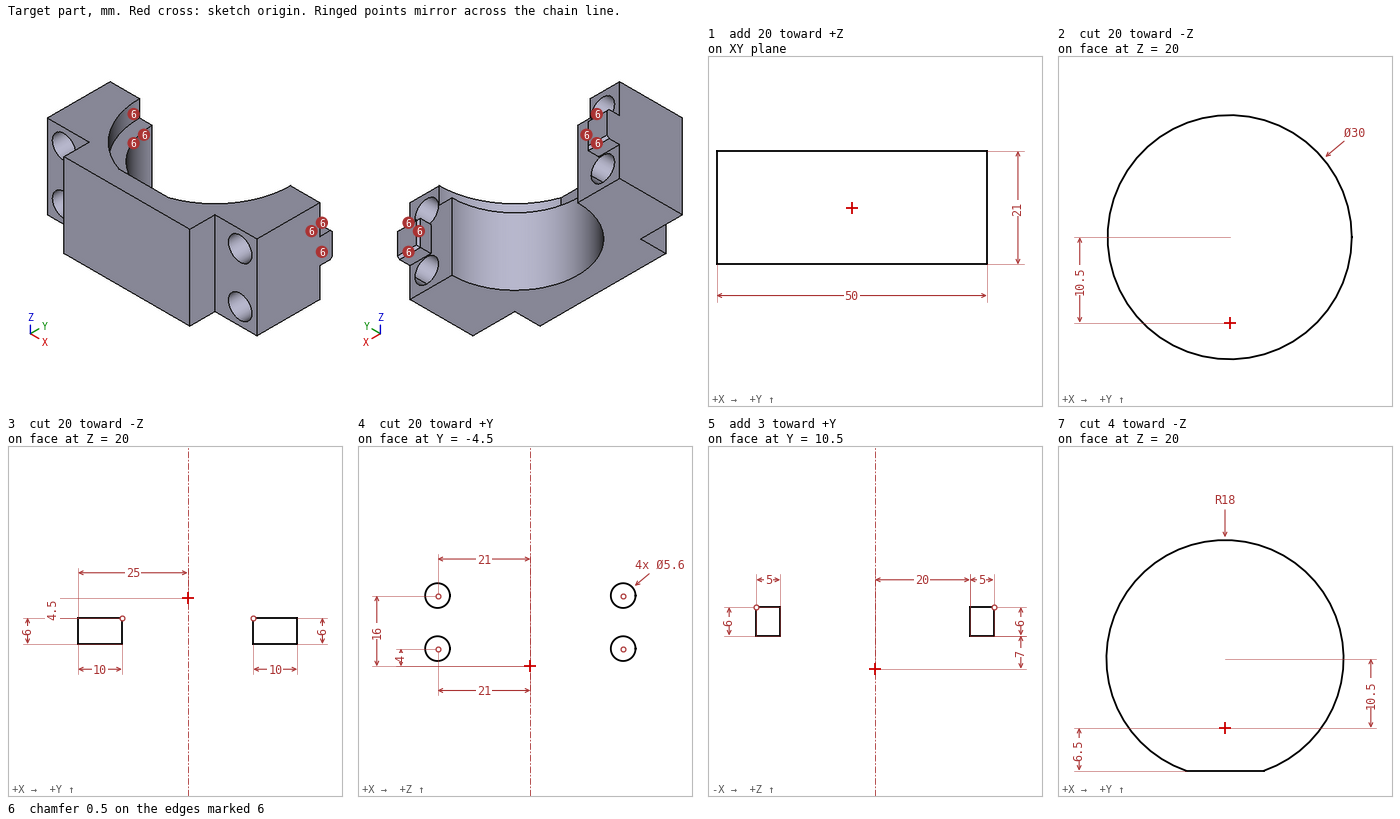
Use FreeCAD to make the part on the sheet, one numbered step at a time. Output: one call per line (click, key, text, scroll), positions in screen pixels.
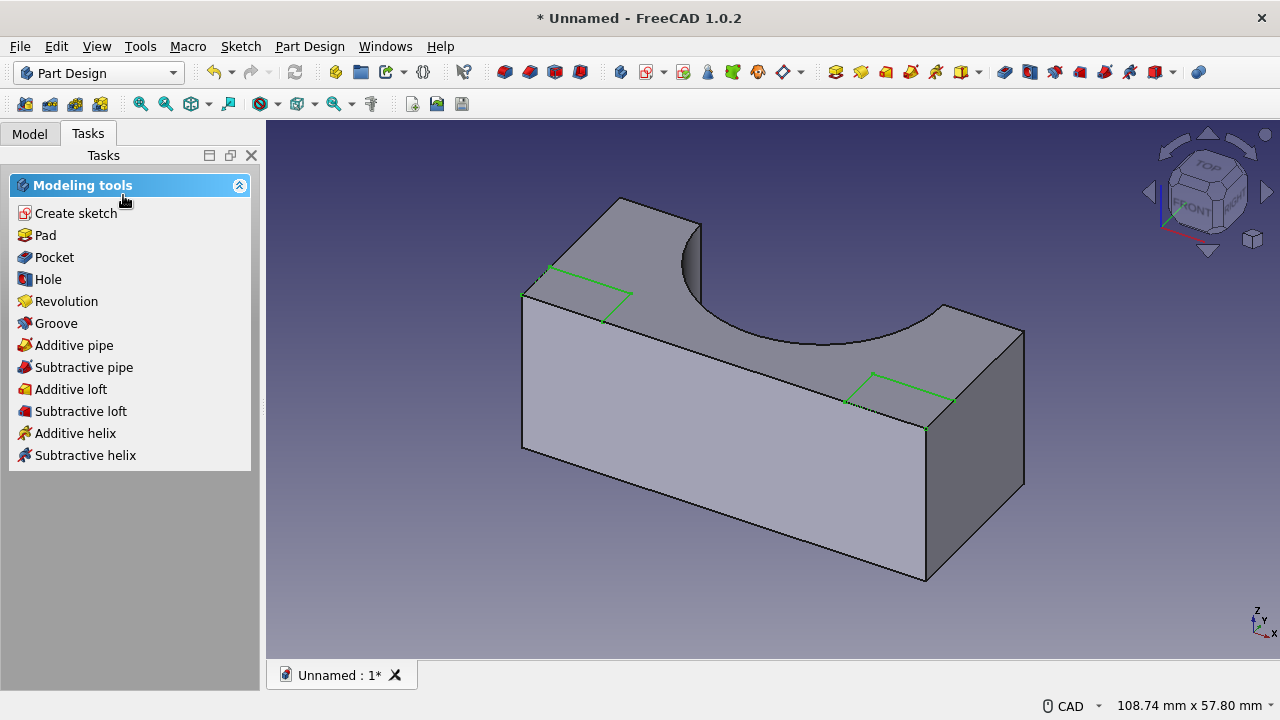
click(1005, 72)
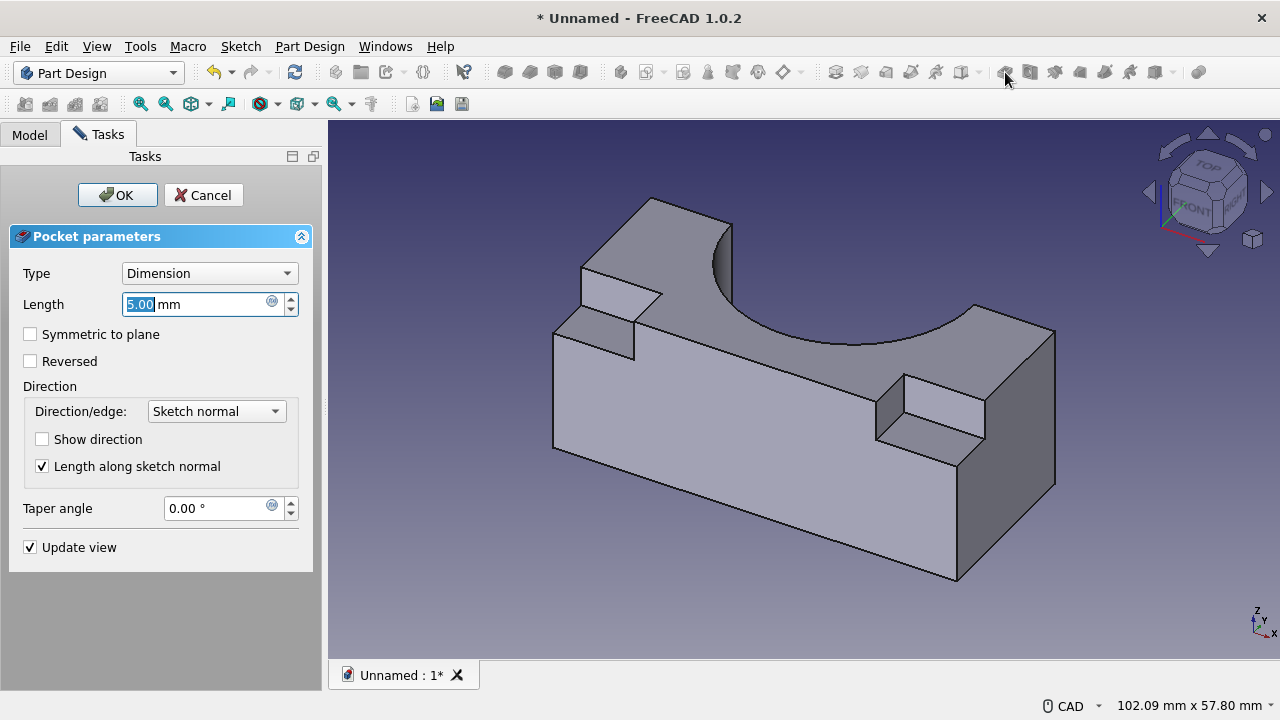
text(20)
key(Tab)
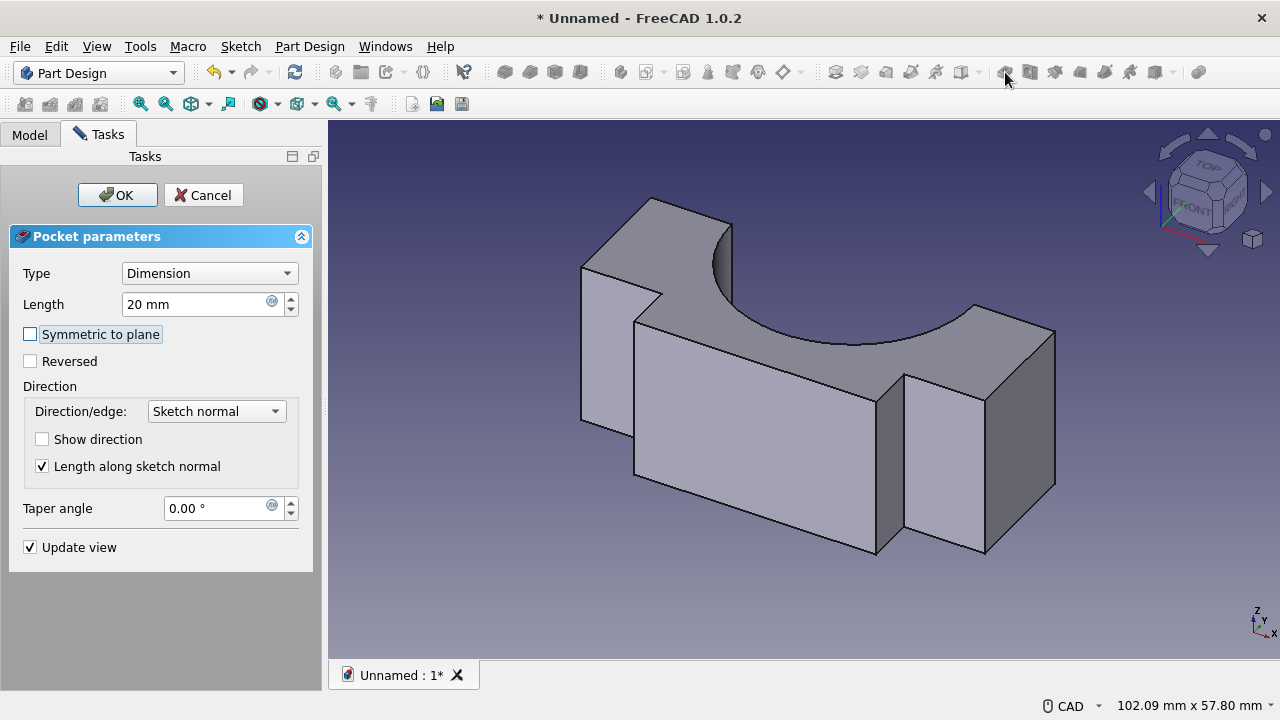
click(118, 195)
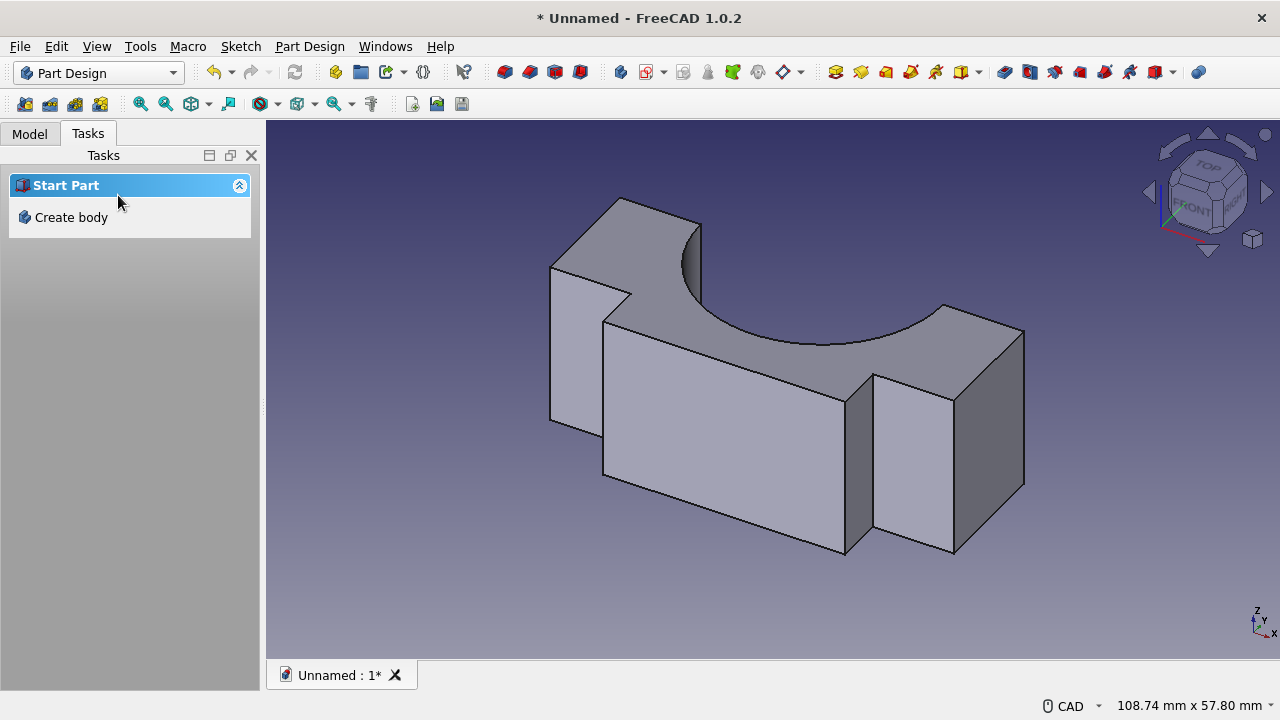
click(591, 334)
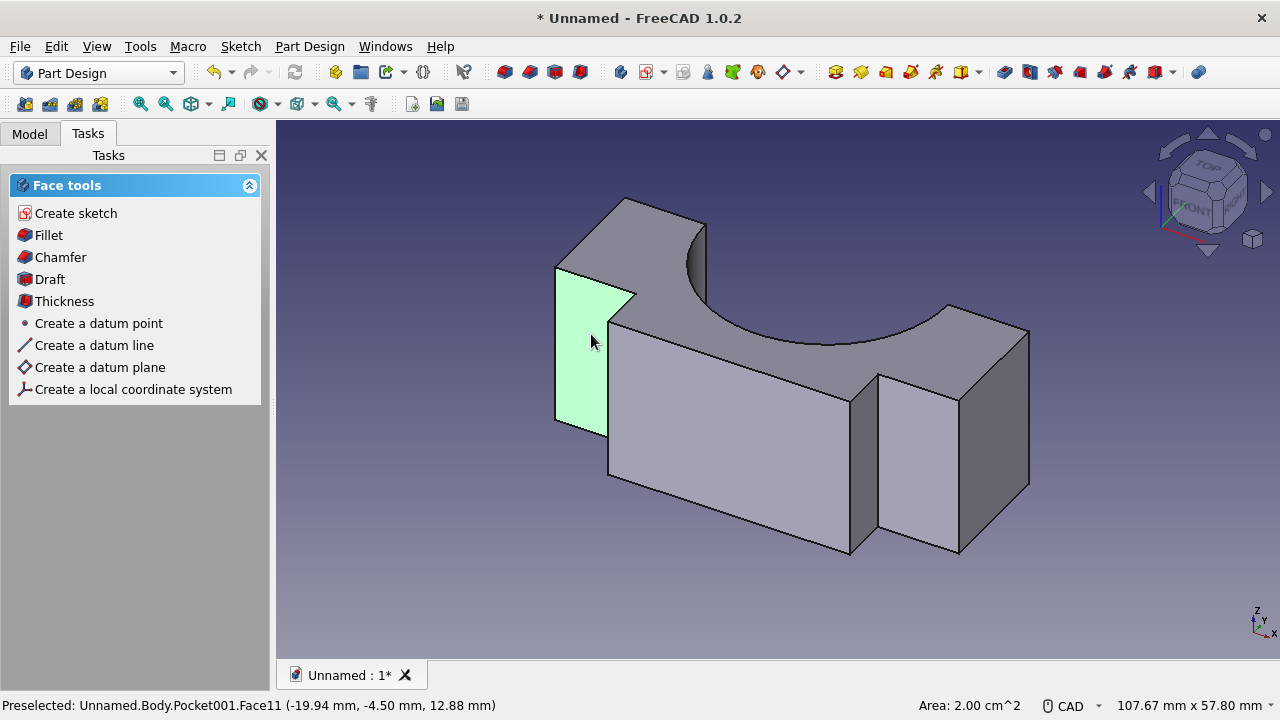
click(646, 72)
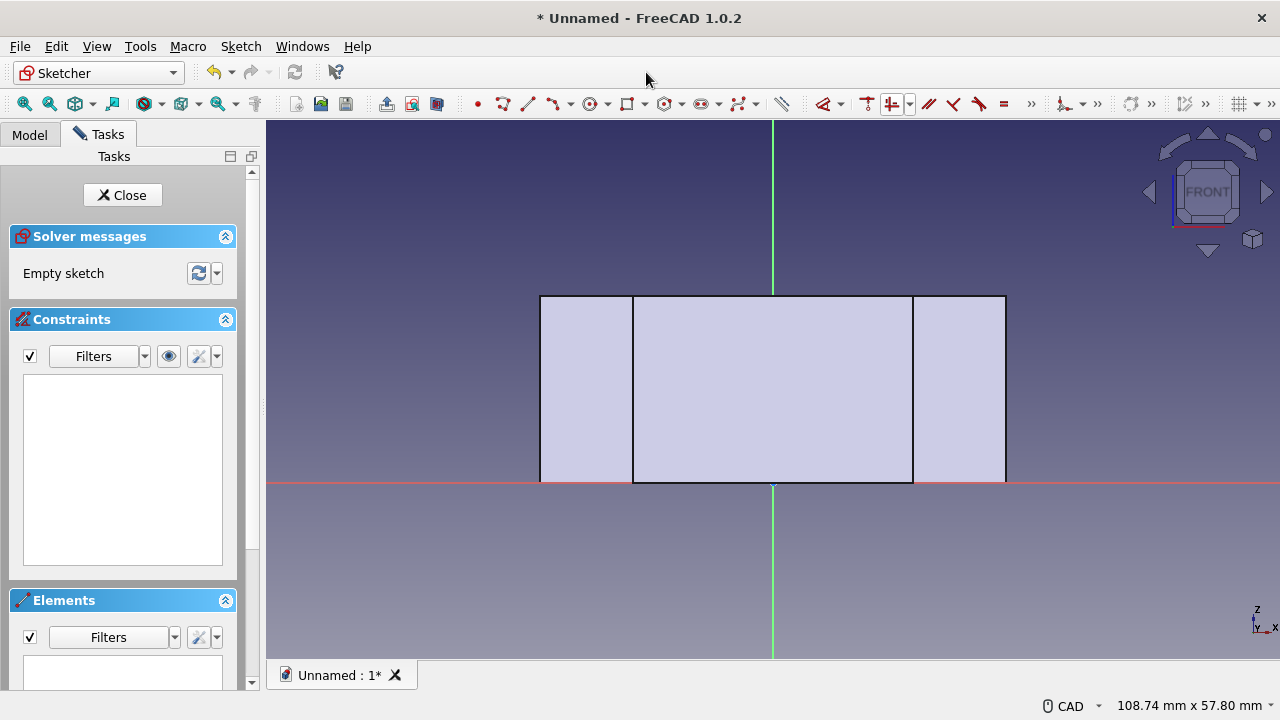
key(q)
key(s)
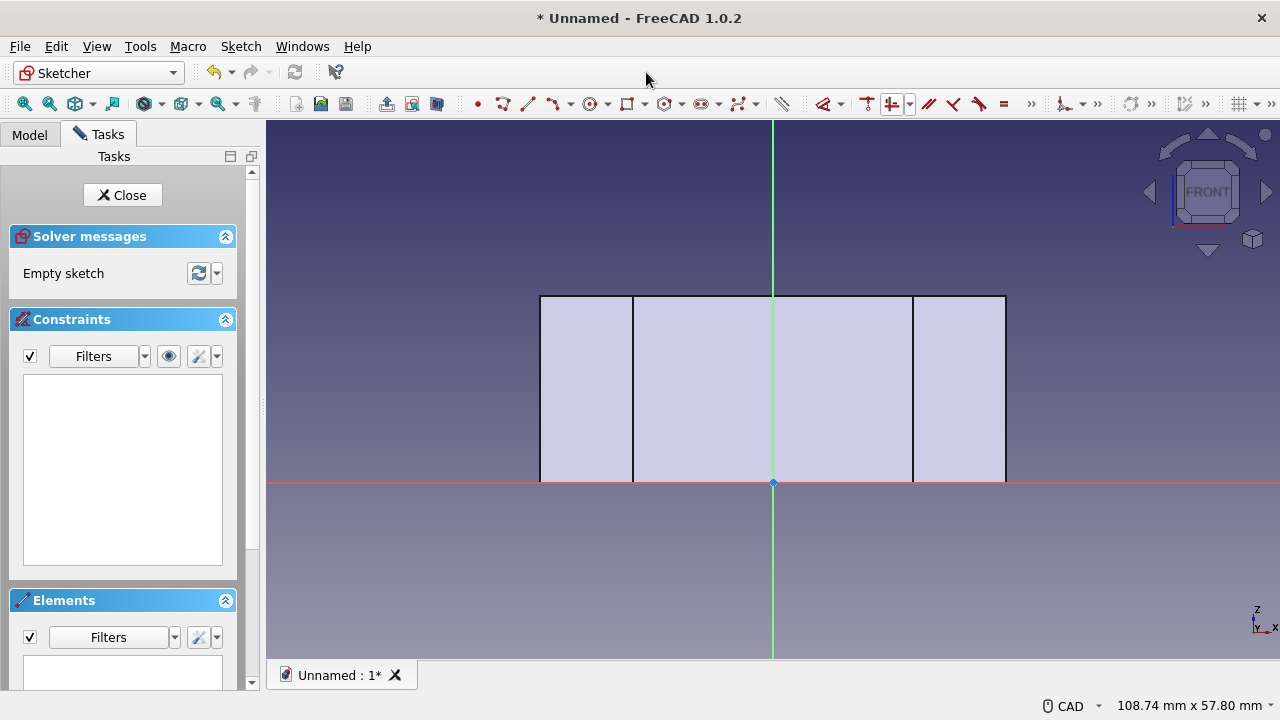
key(g)
key(c)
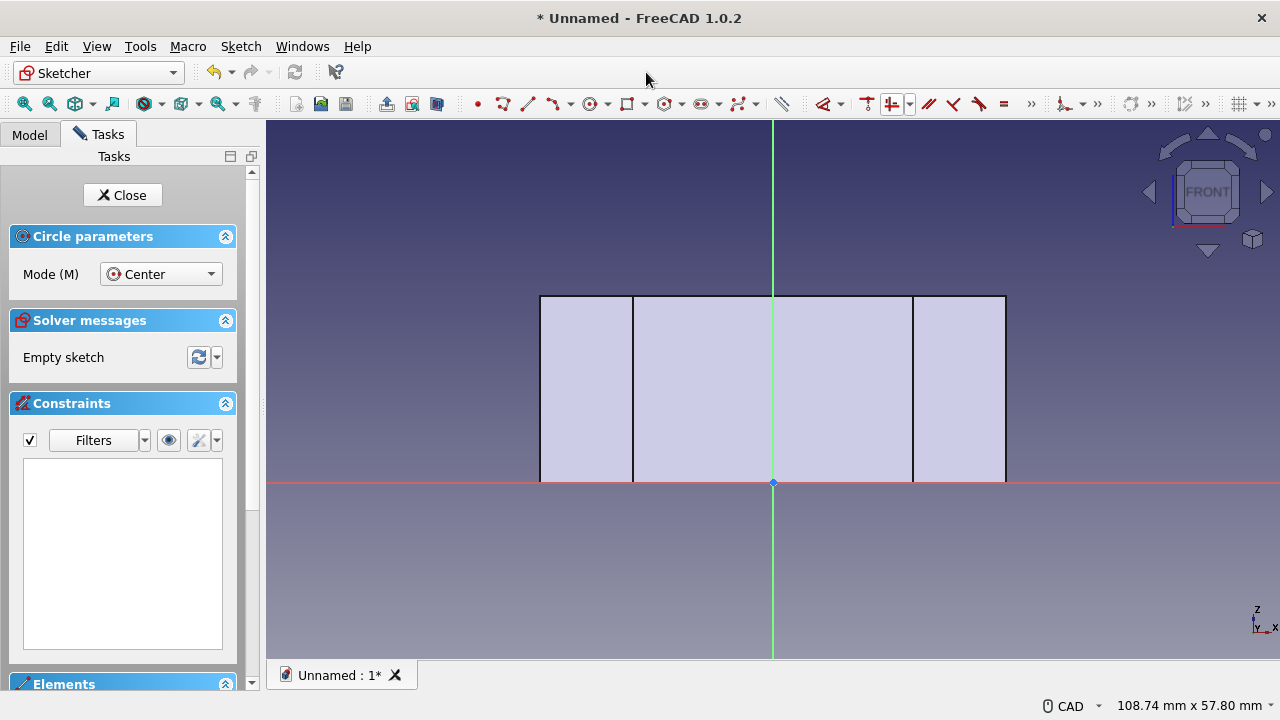
click(577, 334)
move(596, 315)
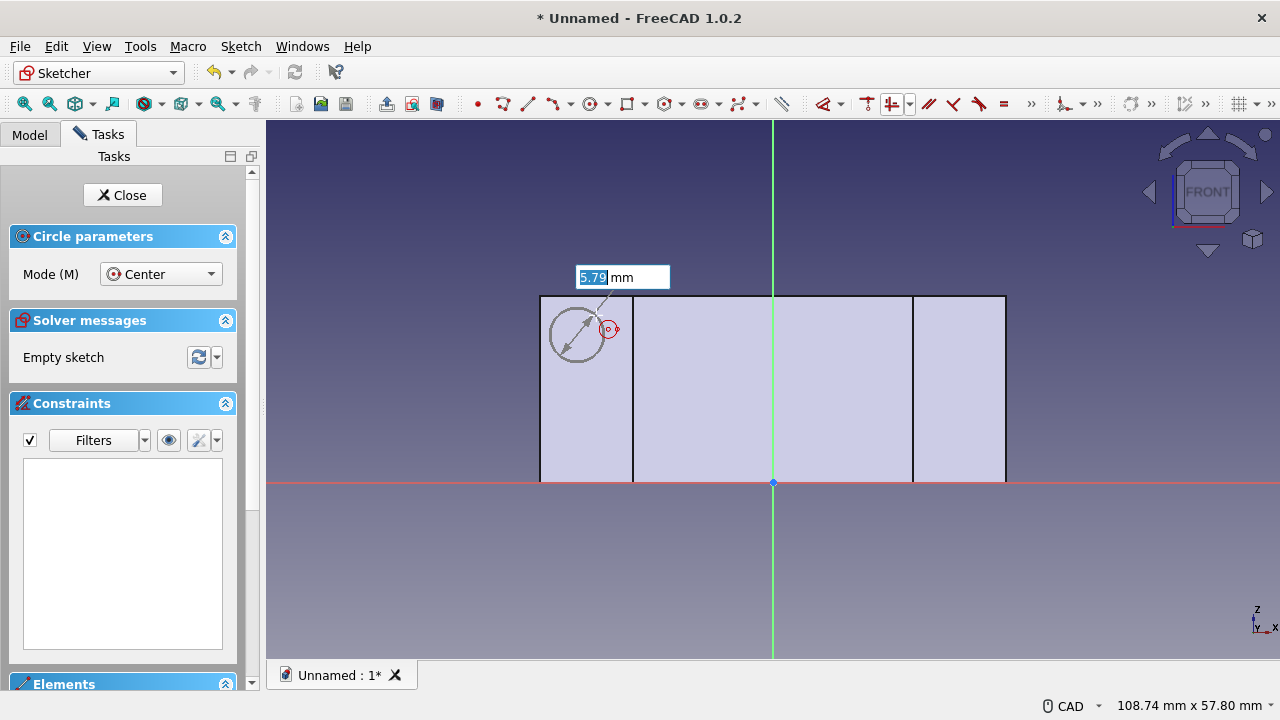
text(5.6)
key(Return)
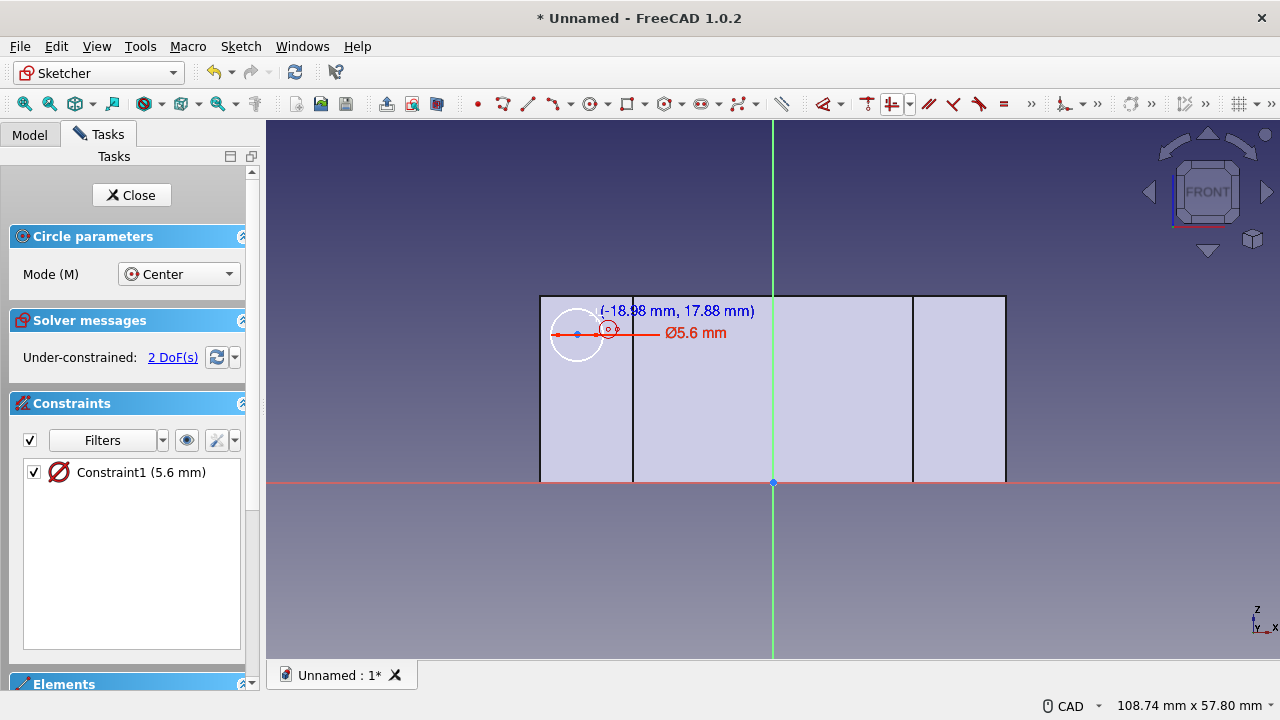
click(577, 445)
move(596, 427)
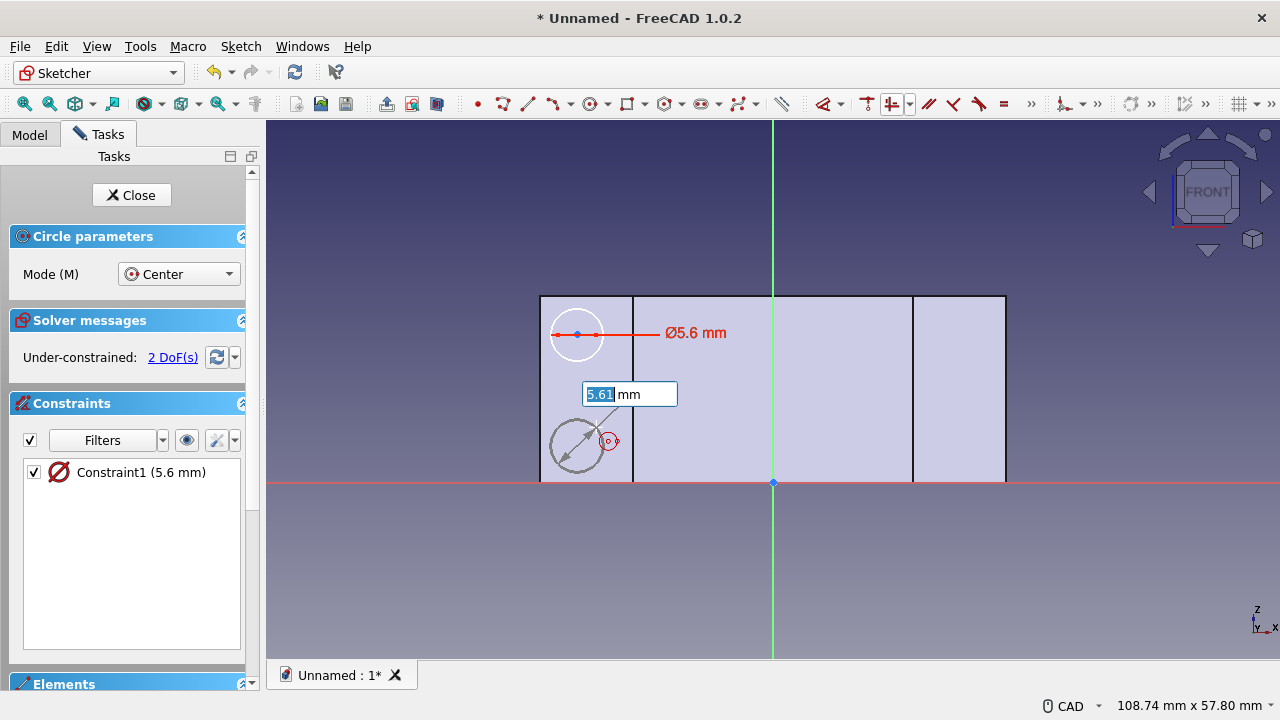
text(5.6)
key(Return)